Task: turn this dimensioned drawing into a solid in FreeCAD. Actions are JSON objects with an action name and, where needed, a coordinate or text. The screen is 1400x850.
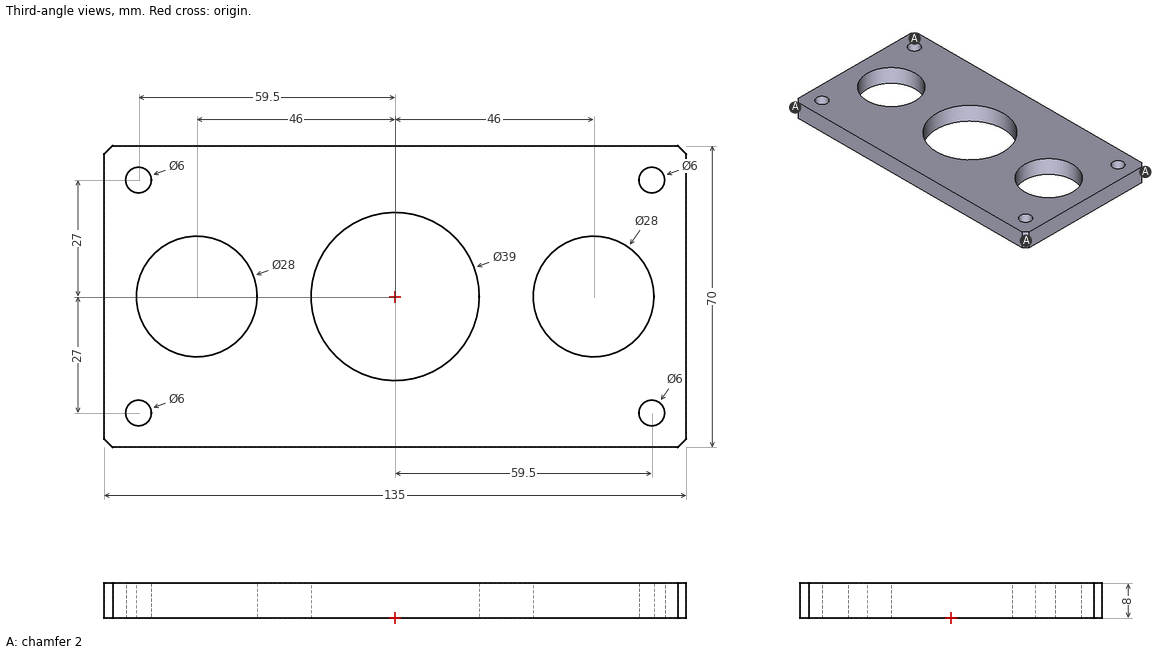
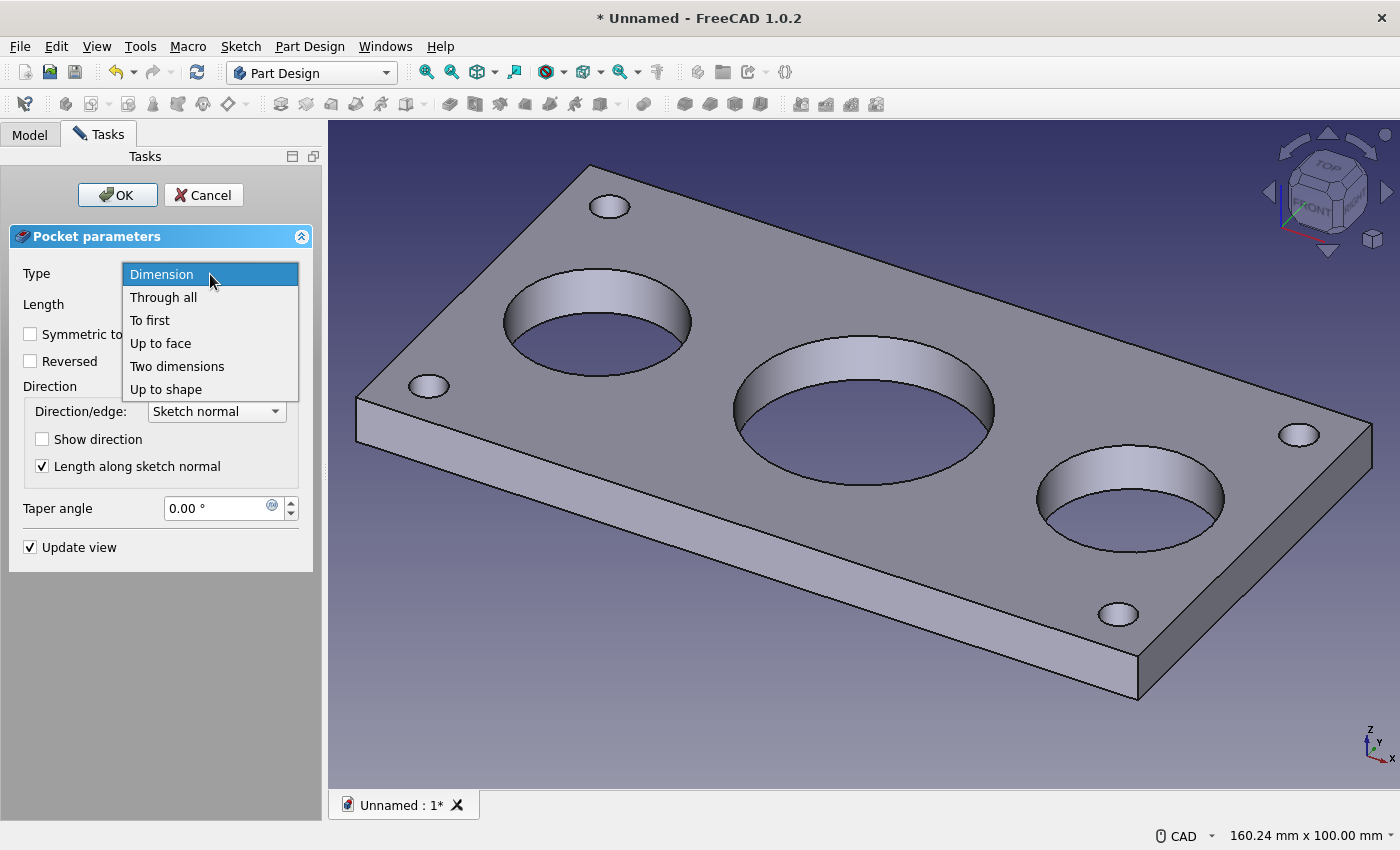
{"action": "left_click", "coordinate": [208, 320]}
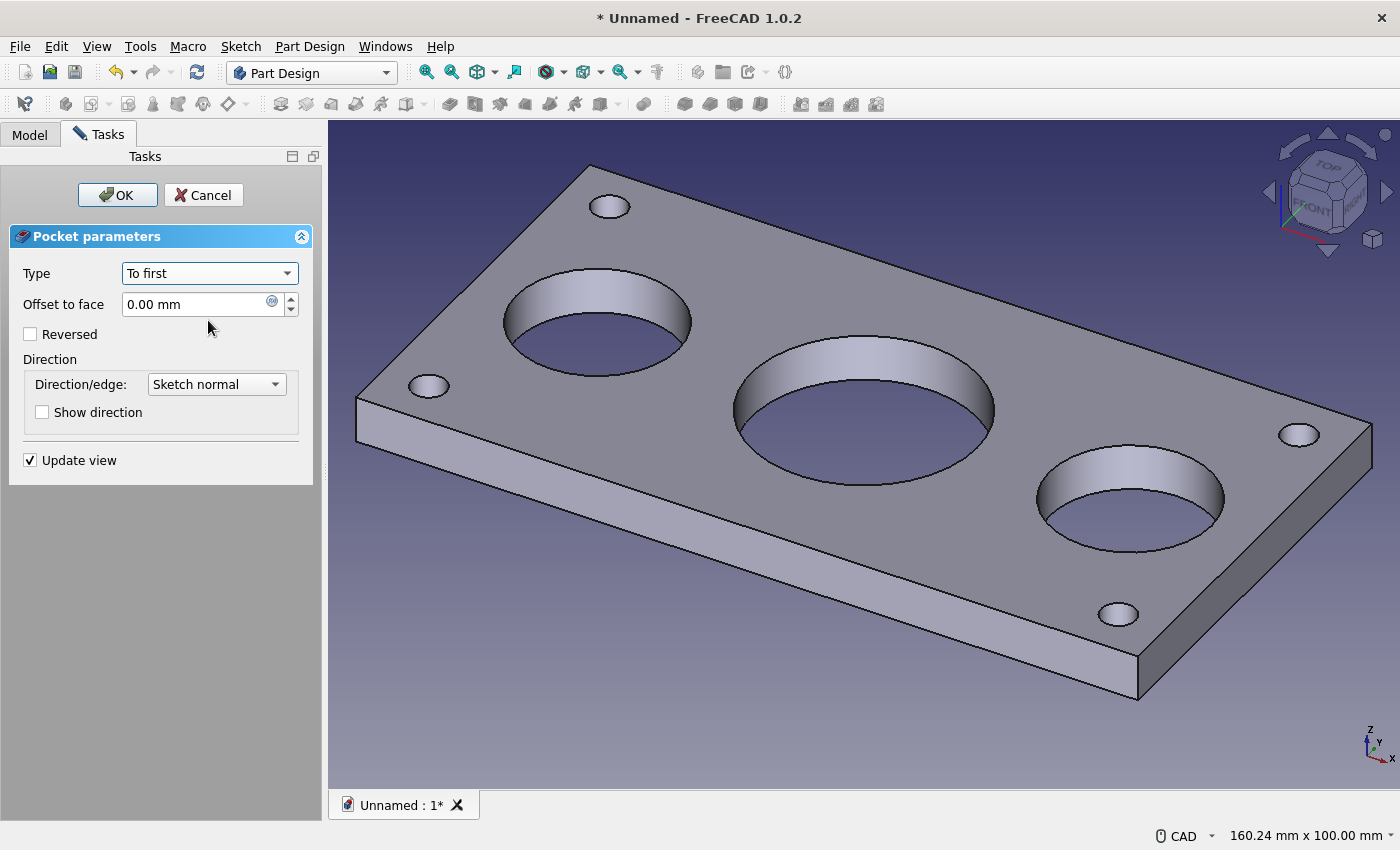
{"action": "left_click", "coordinate": [118, 195]}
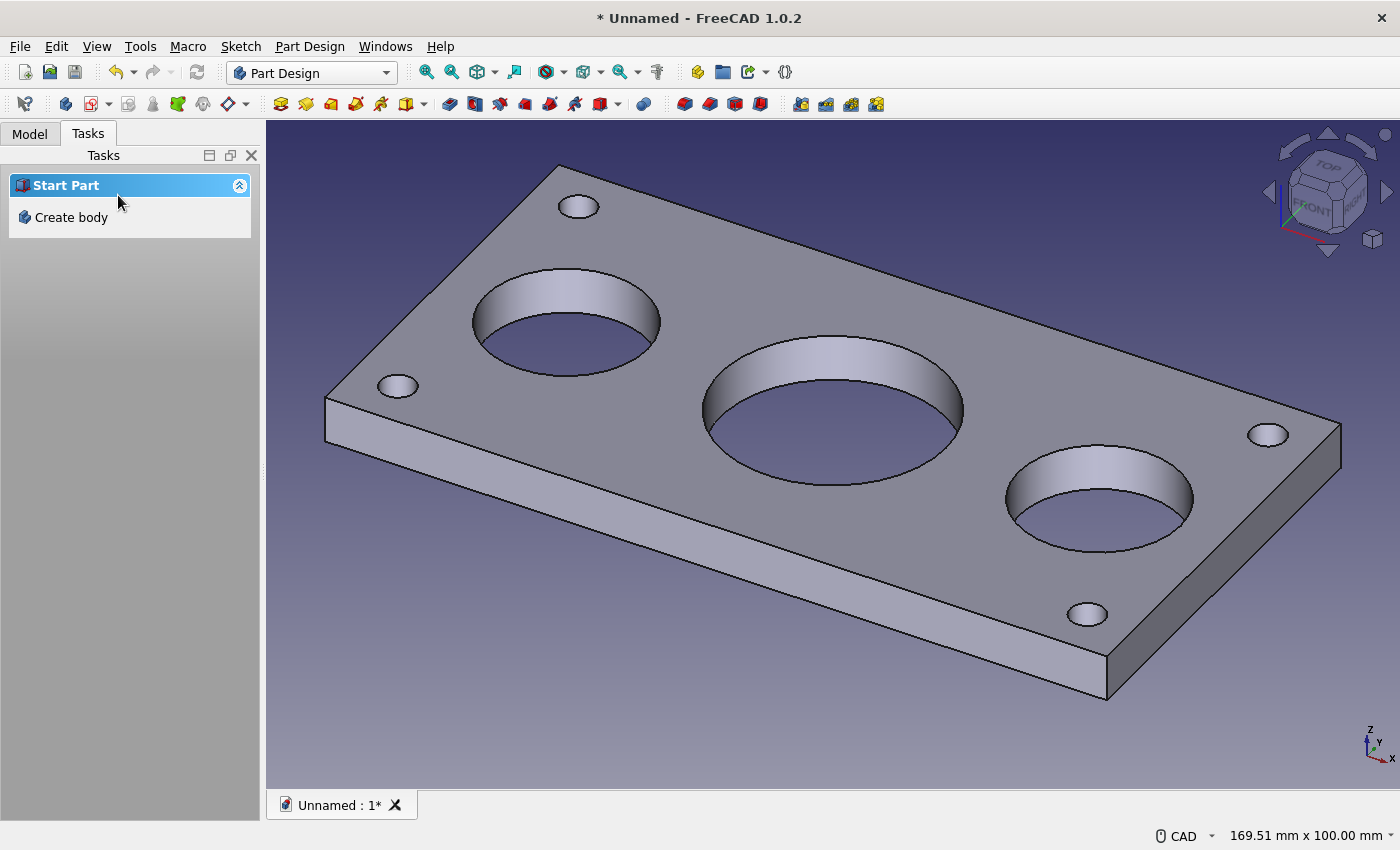
{"action": "left_click", "coordinate": [1107, 677]}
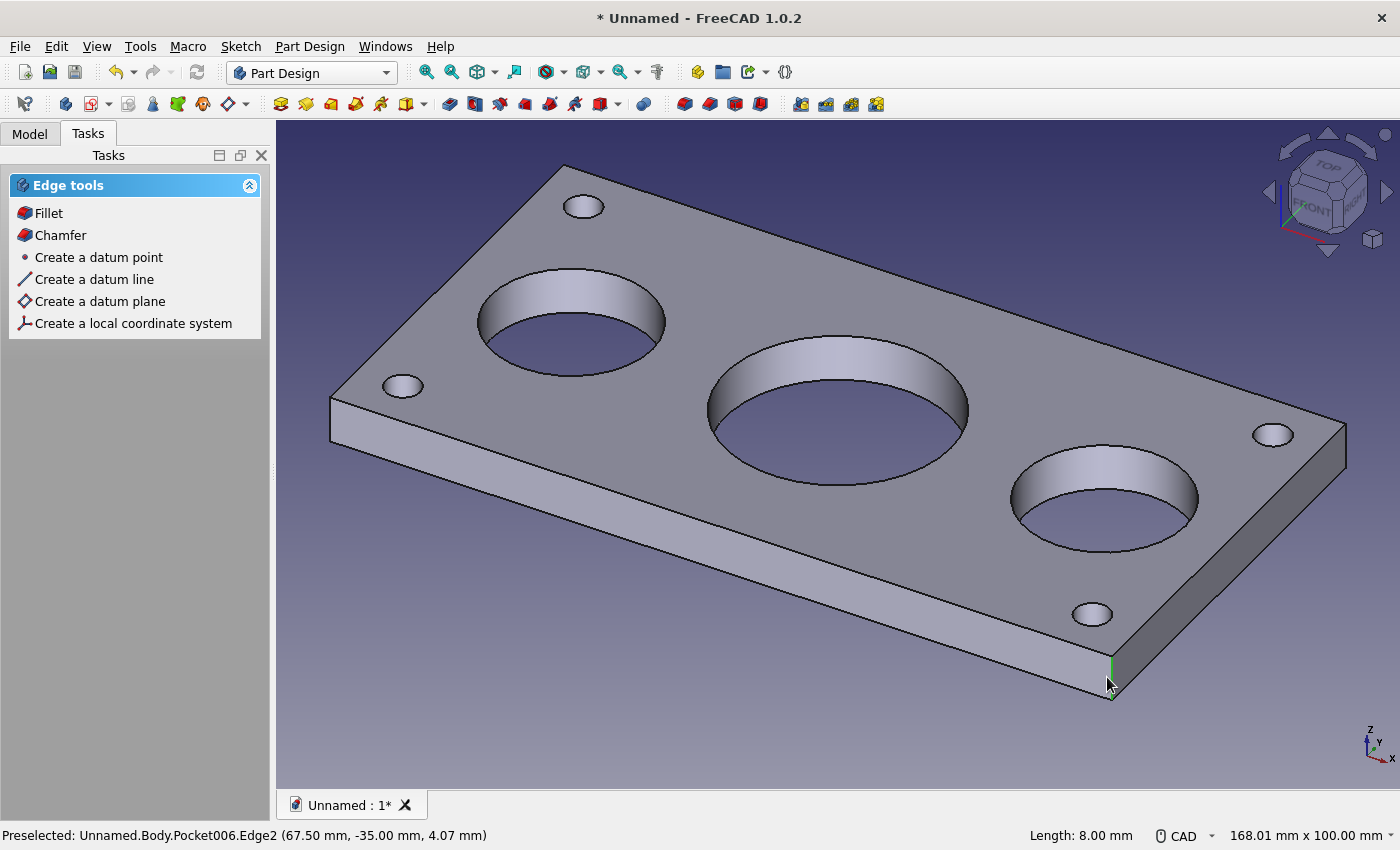
{"action": "key", "text": "0"}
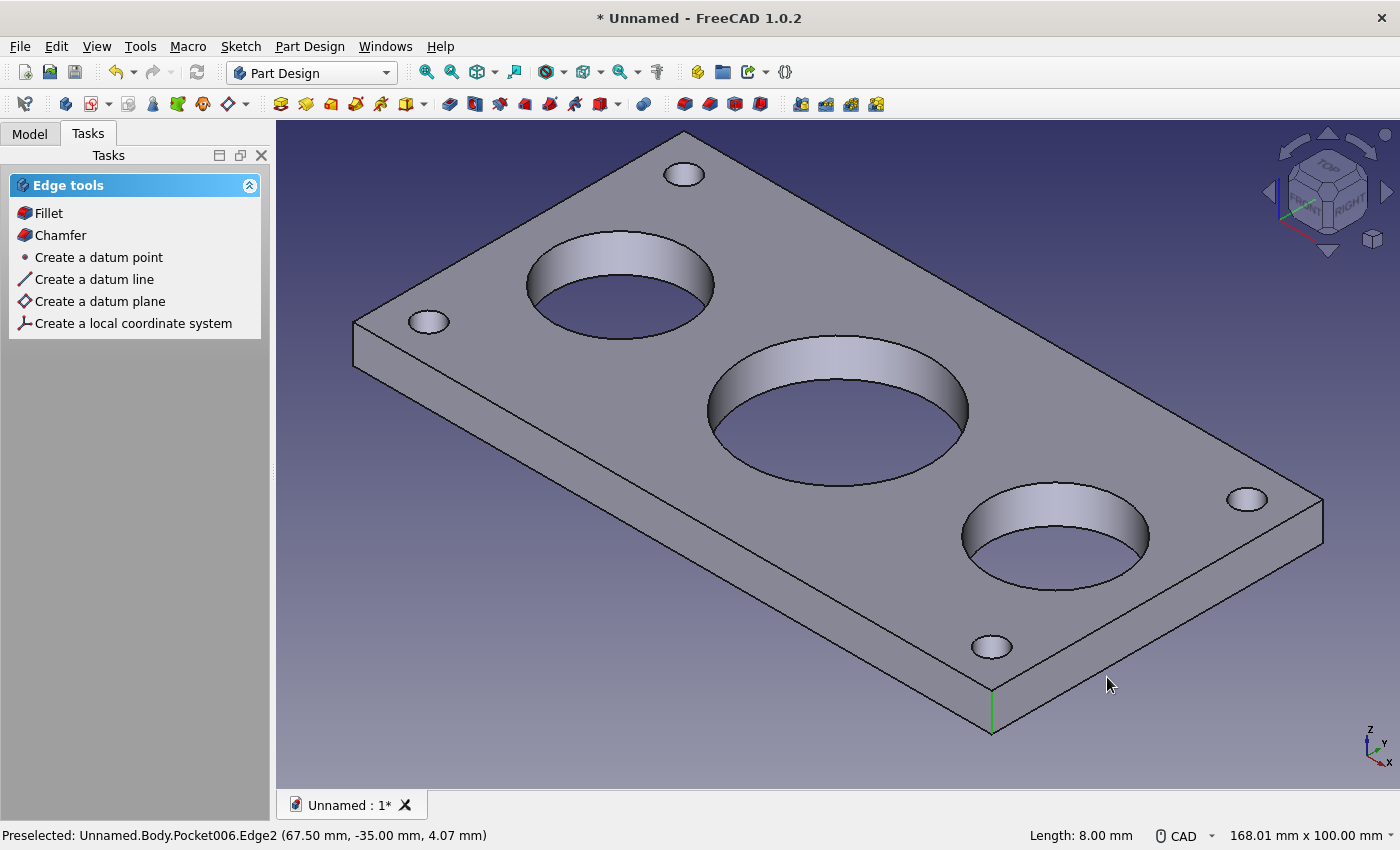
{"action": "key", "text": "2"}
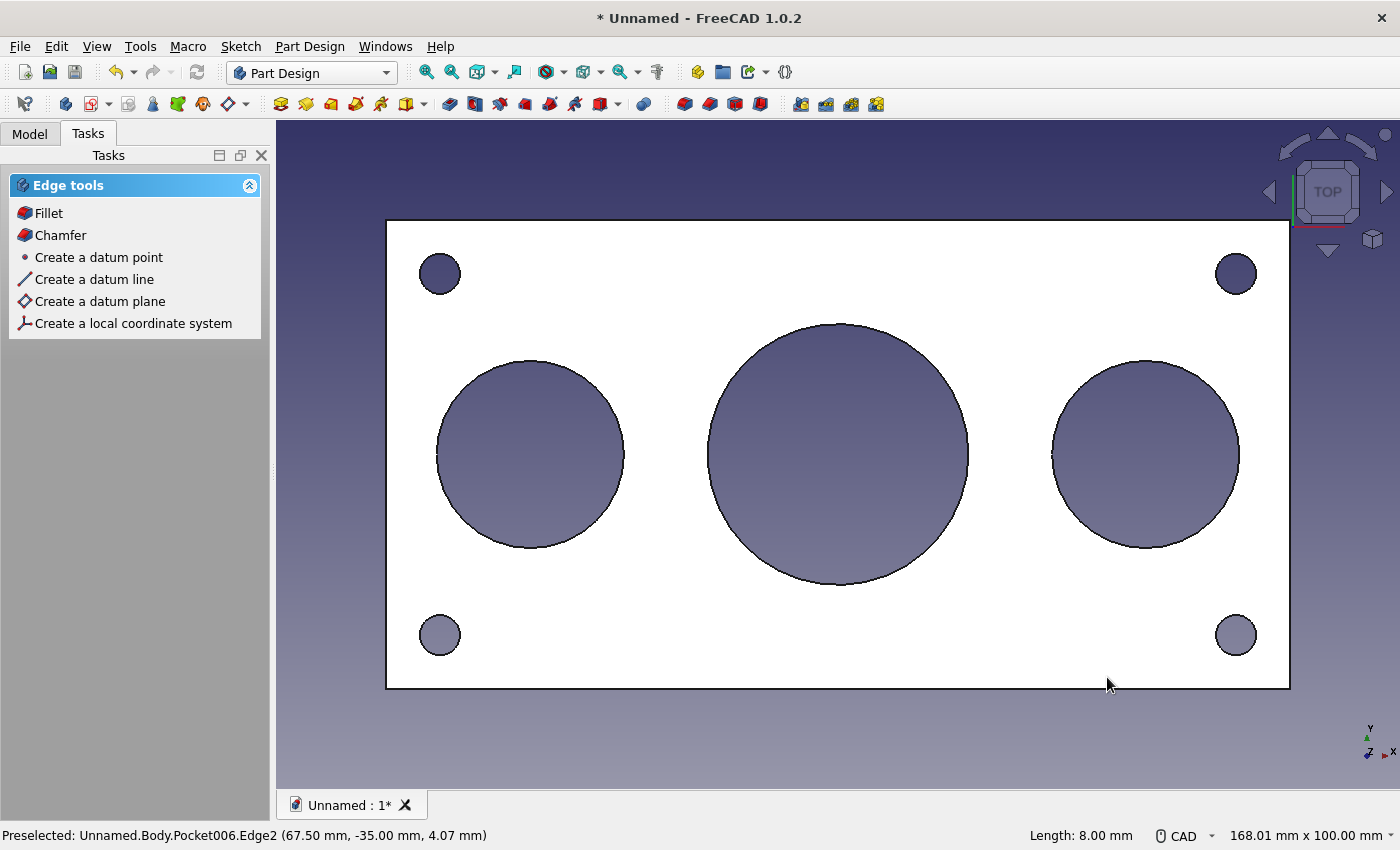
{"action": "key", "text": "1"}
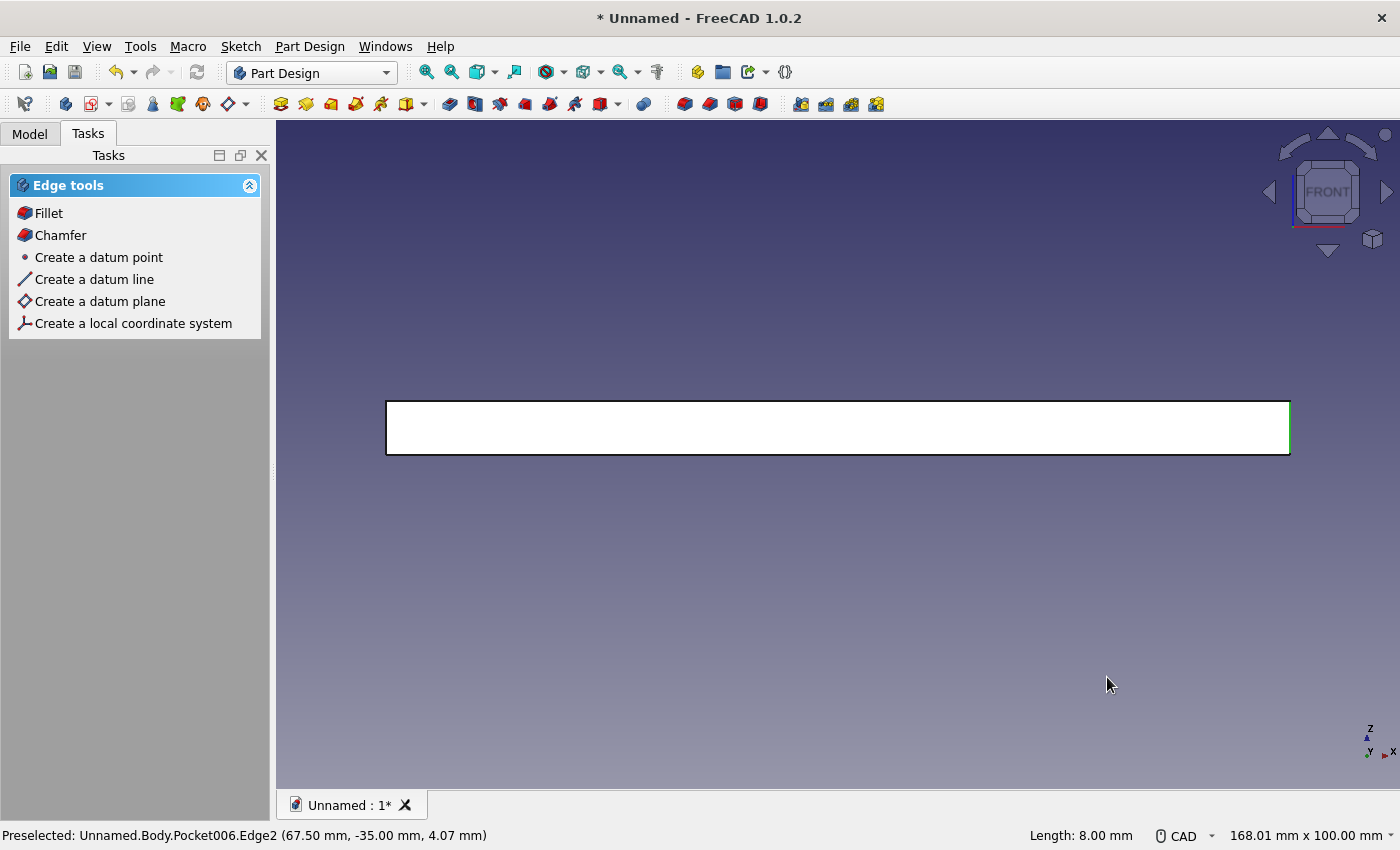
{"action": "left_click", "coordinate": [386, 427], "text": "ctrl"}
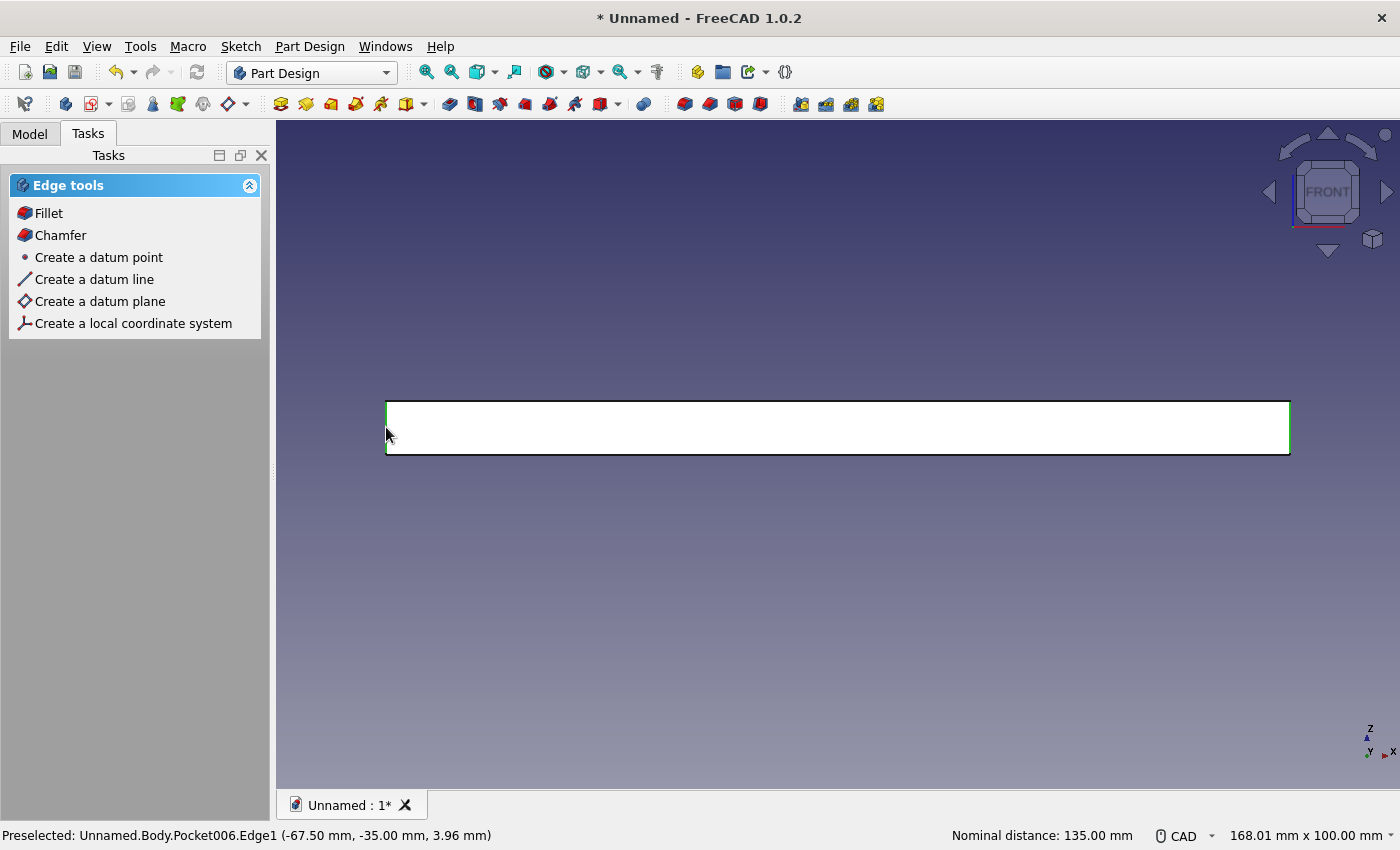
{"action": "key", "text": "3"}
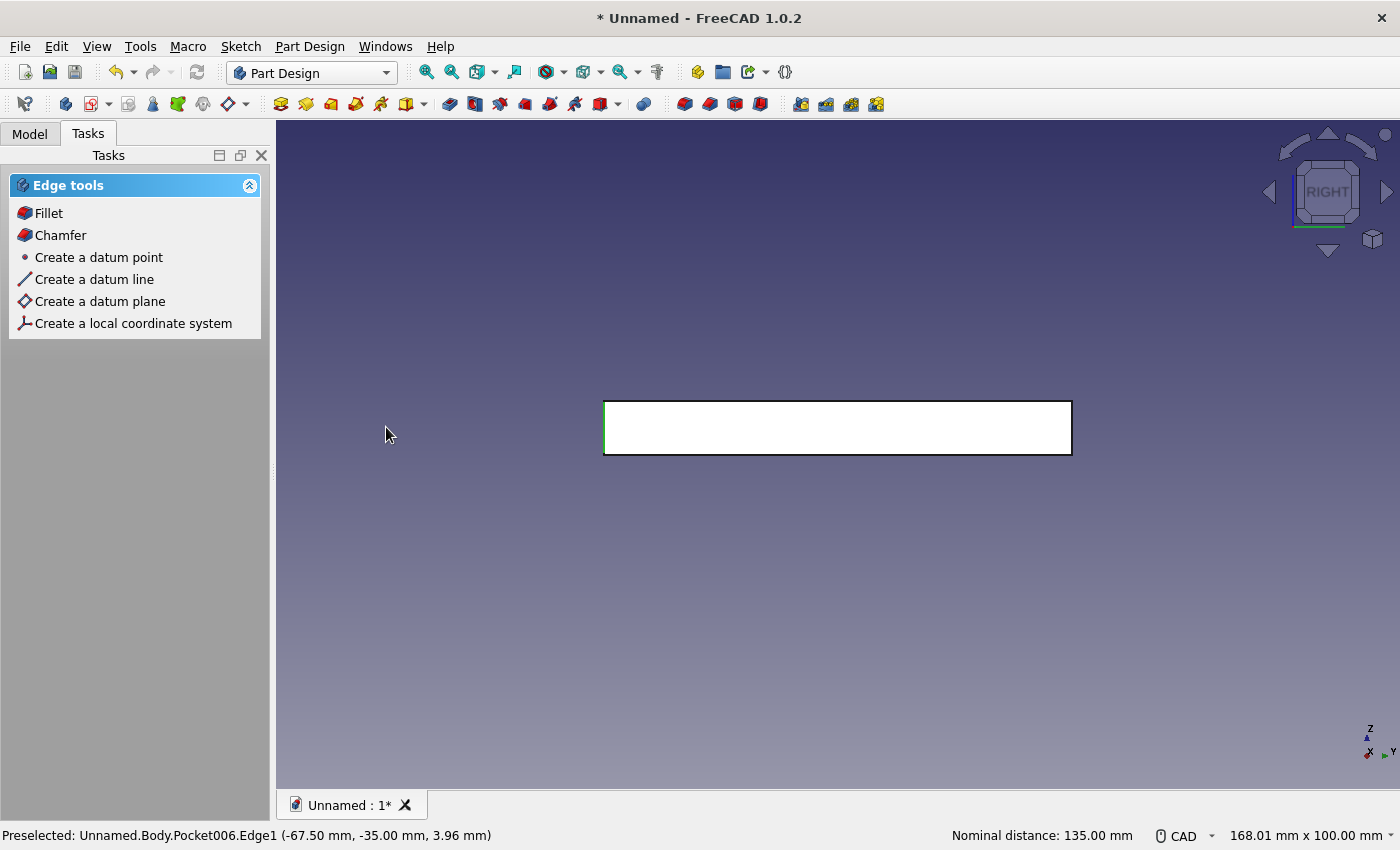
{"action": "key", "text": "v f"}